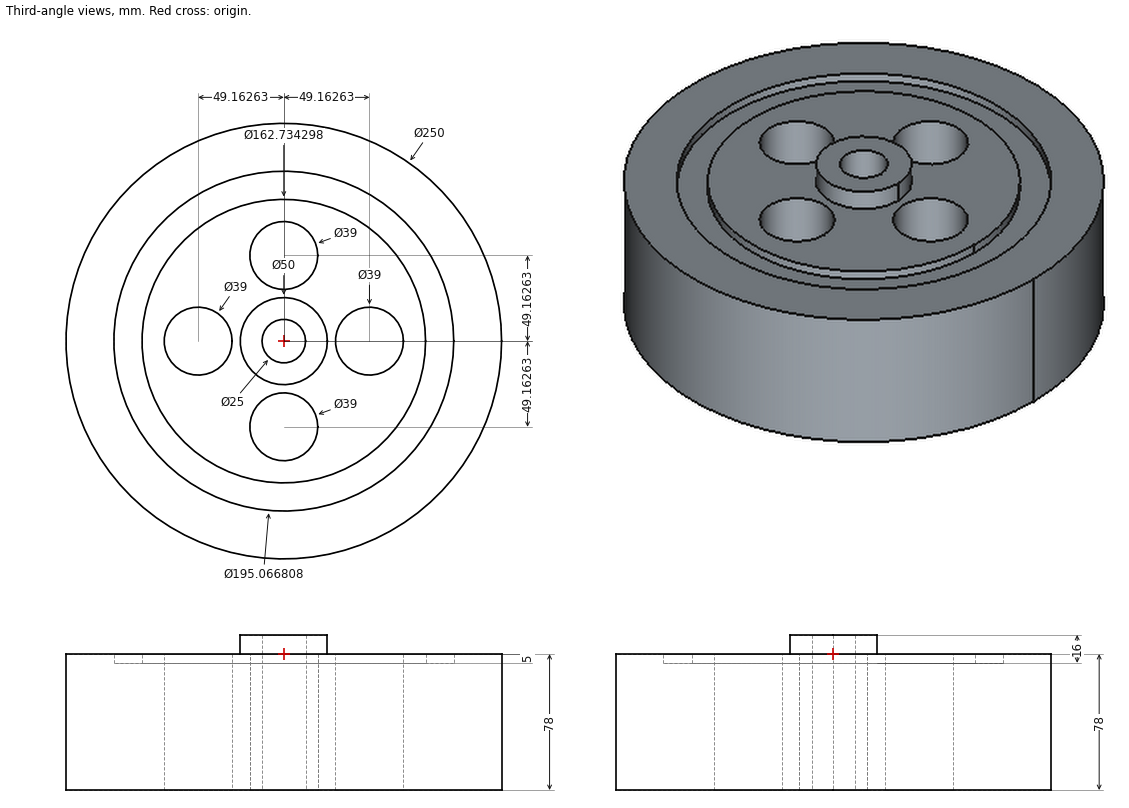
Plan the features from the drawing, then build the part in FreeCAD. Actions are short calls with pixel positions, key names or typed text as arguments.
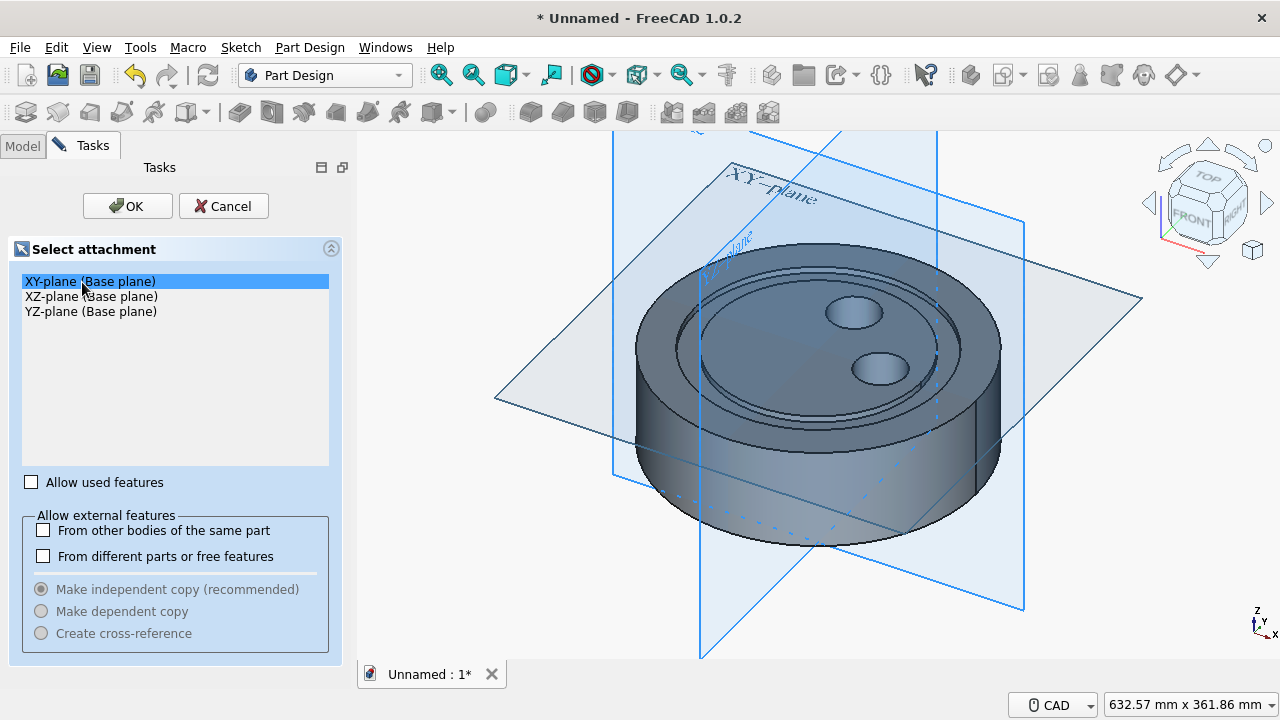
click(128, 206)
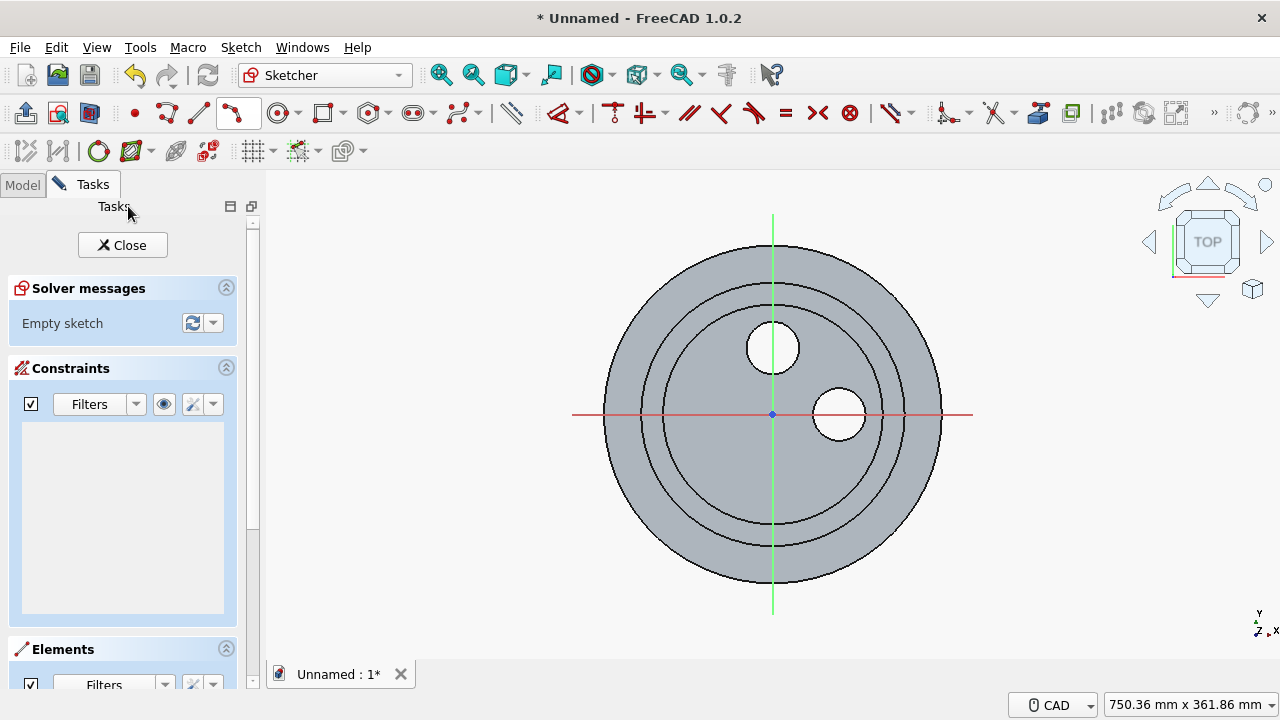
scroll(802, 481, up, 6)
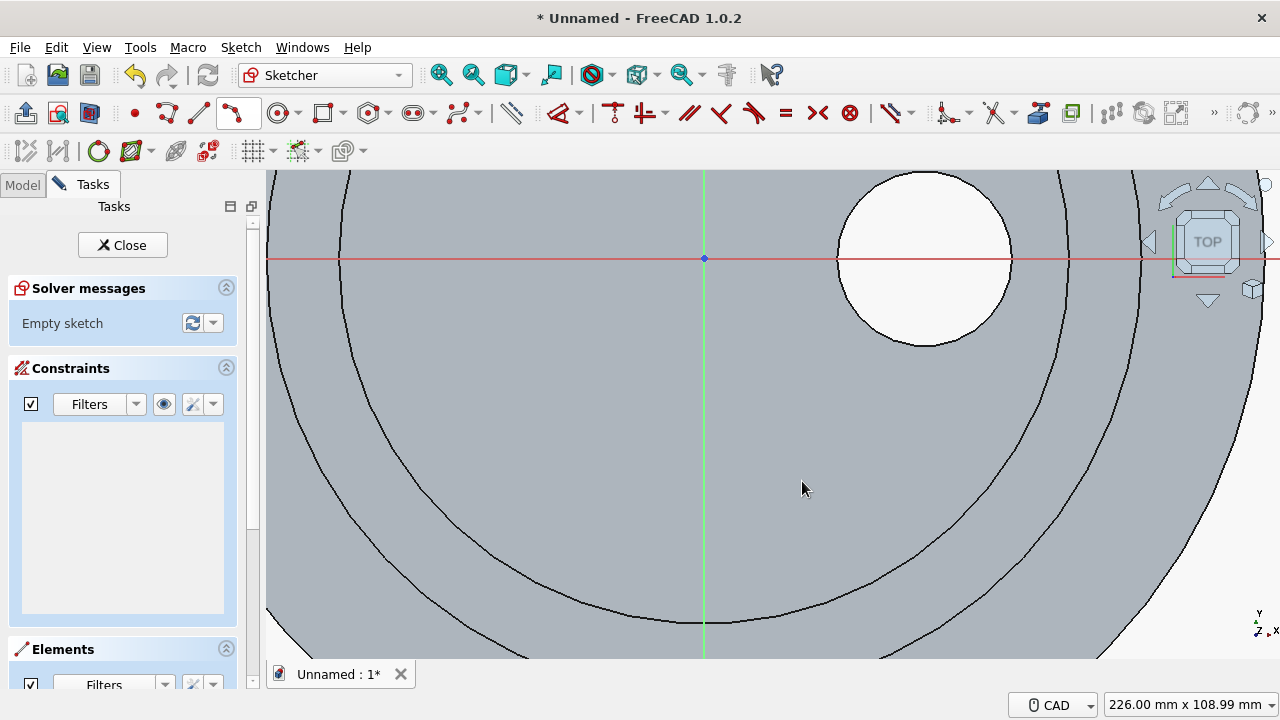
key(g)
key(c)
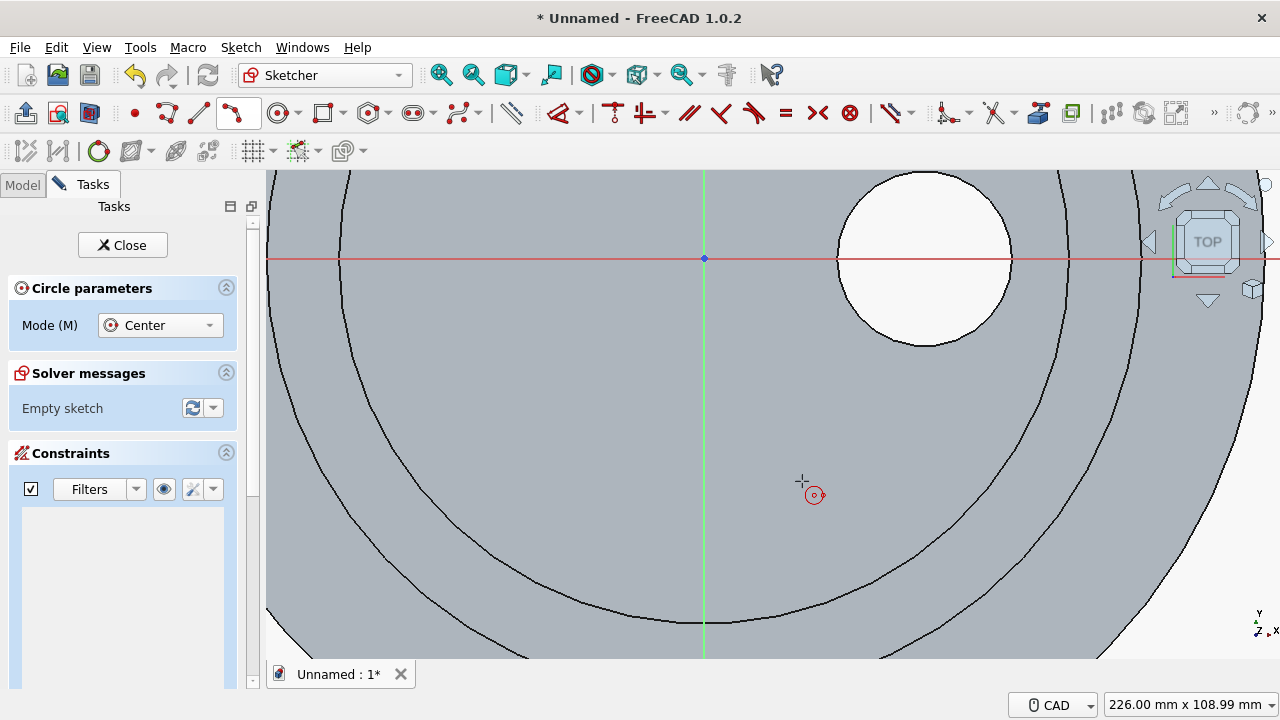
click(704, 479)
move(766, 417)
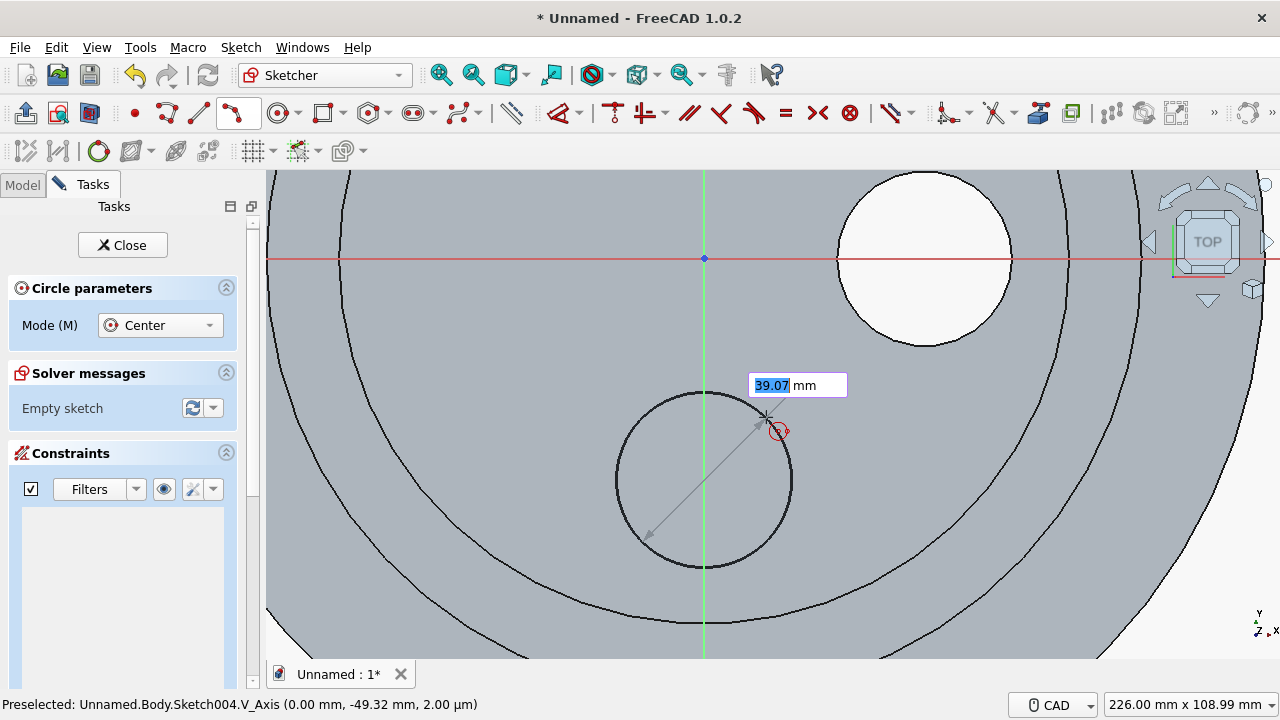
text(39)
key(Return)
key(Escape)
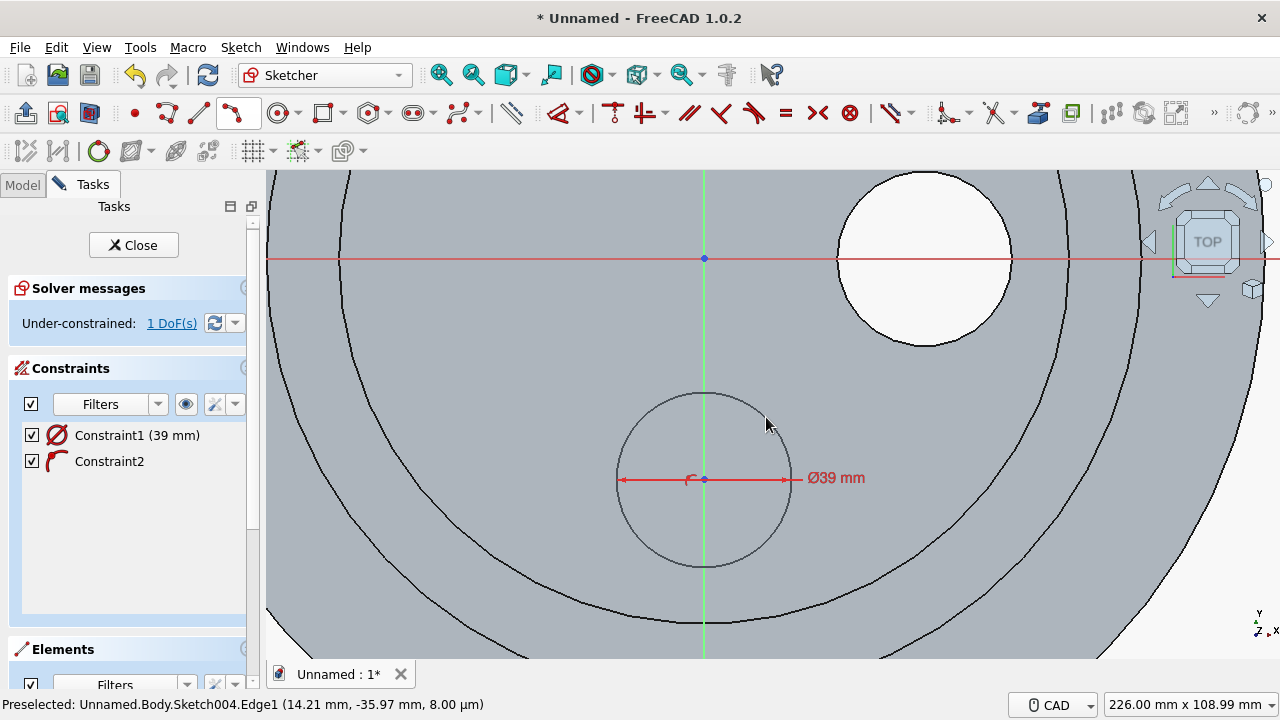
click(558, 114)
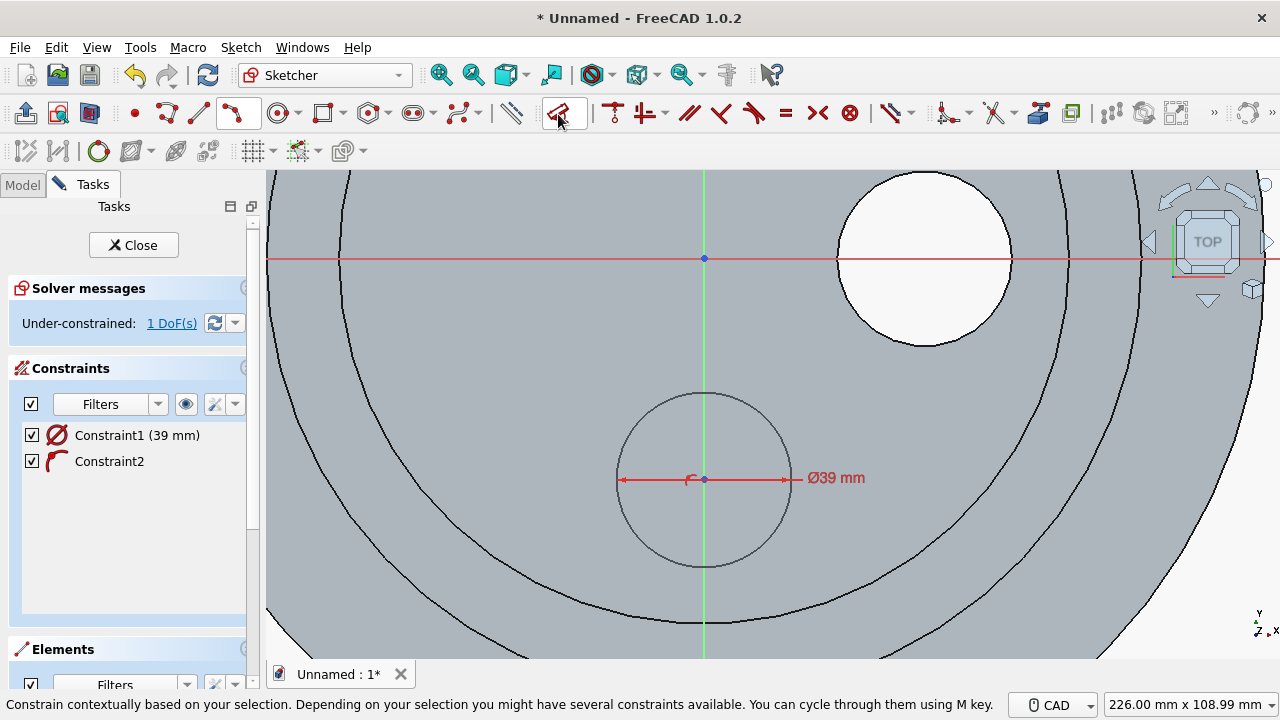
click(704, 480)
click(738, 369)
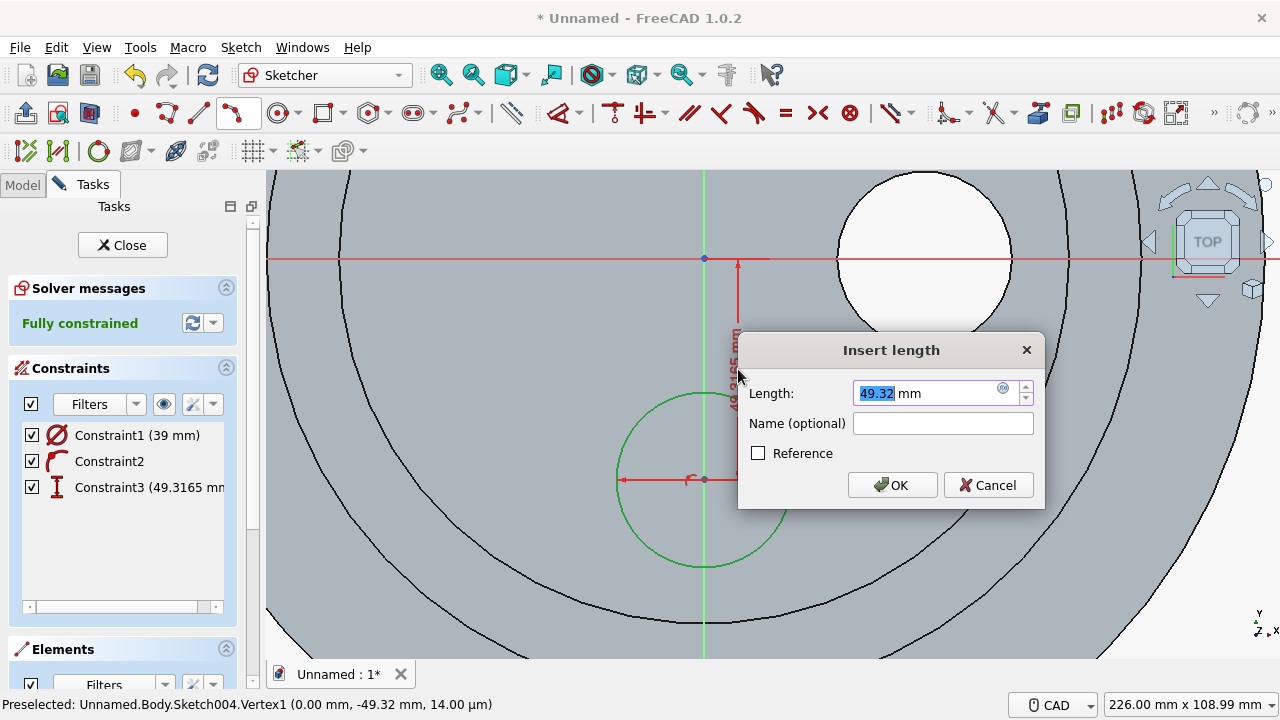
text(49.16263)
key(Return)
key(Escape)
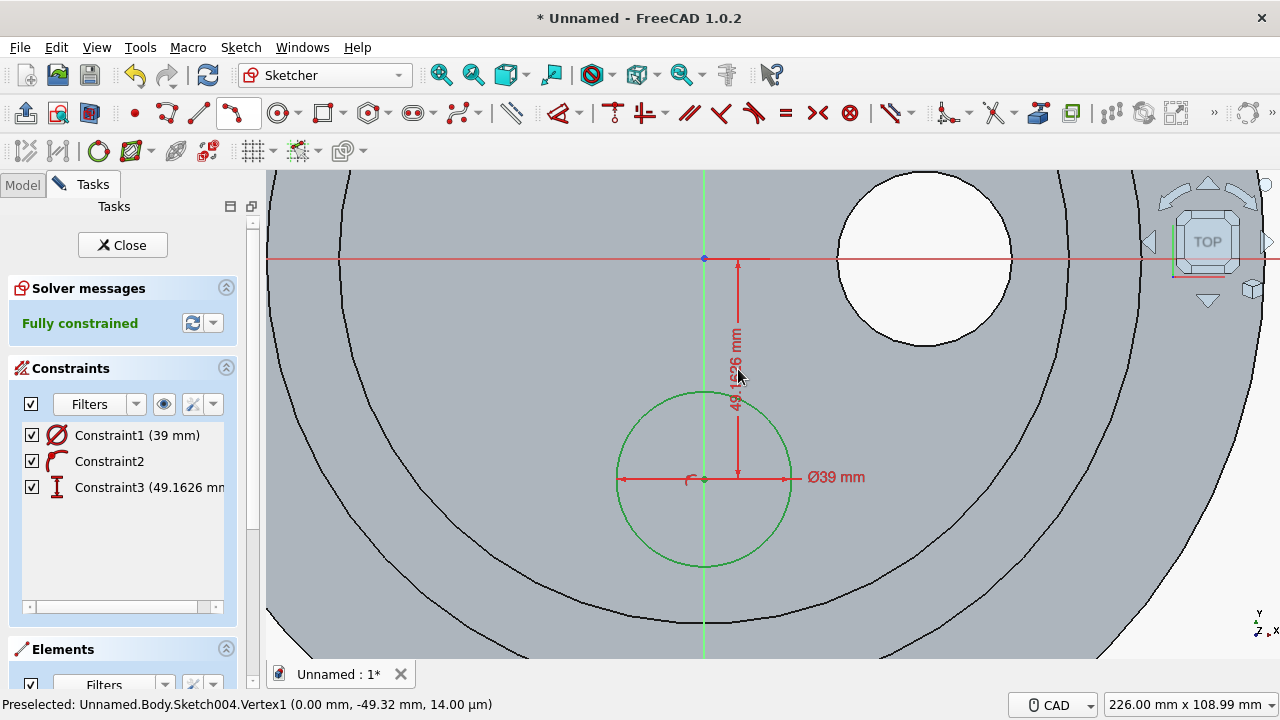
click(123, 245)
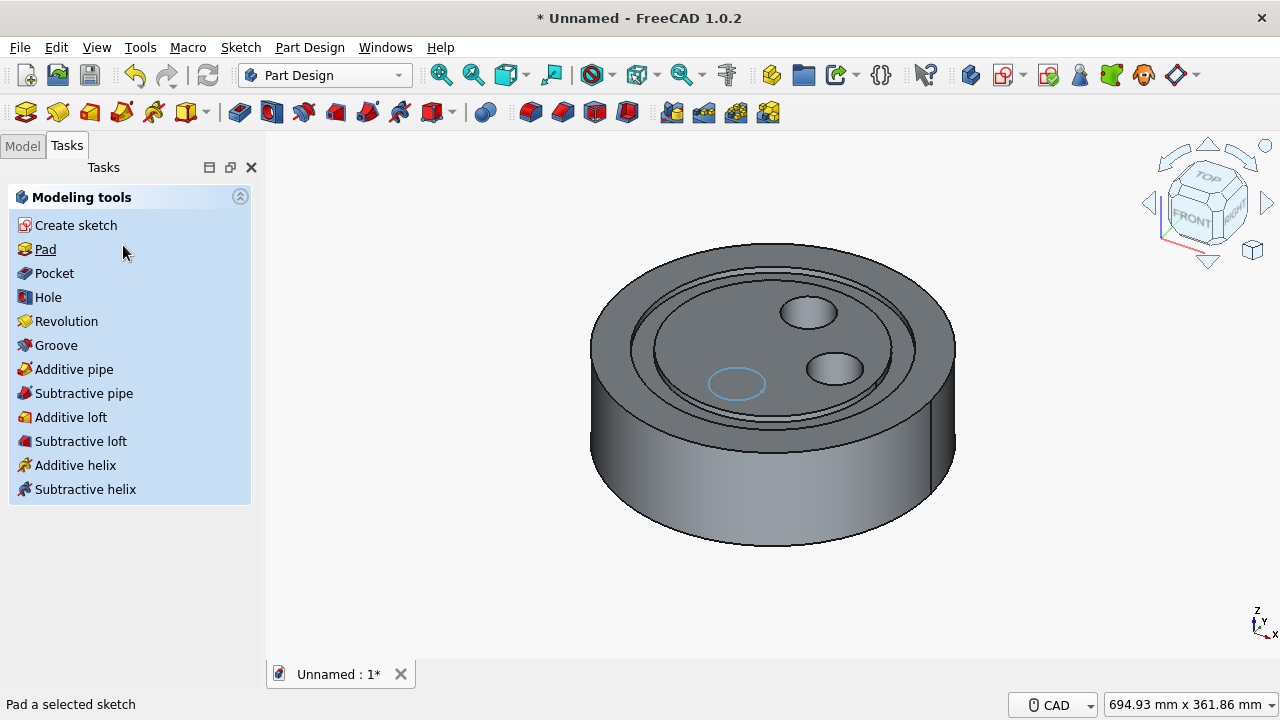
click(240, 112)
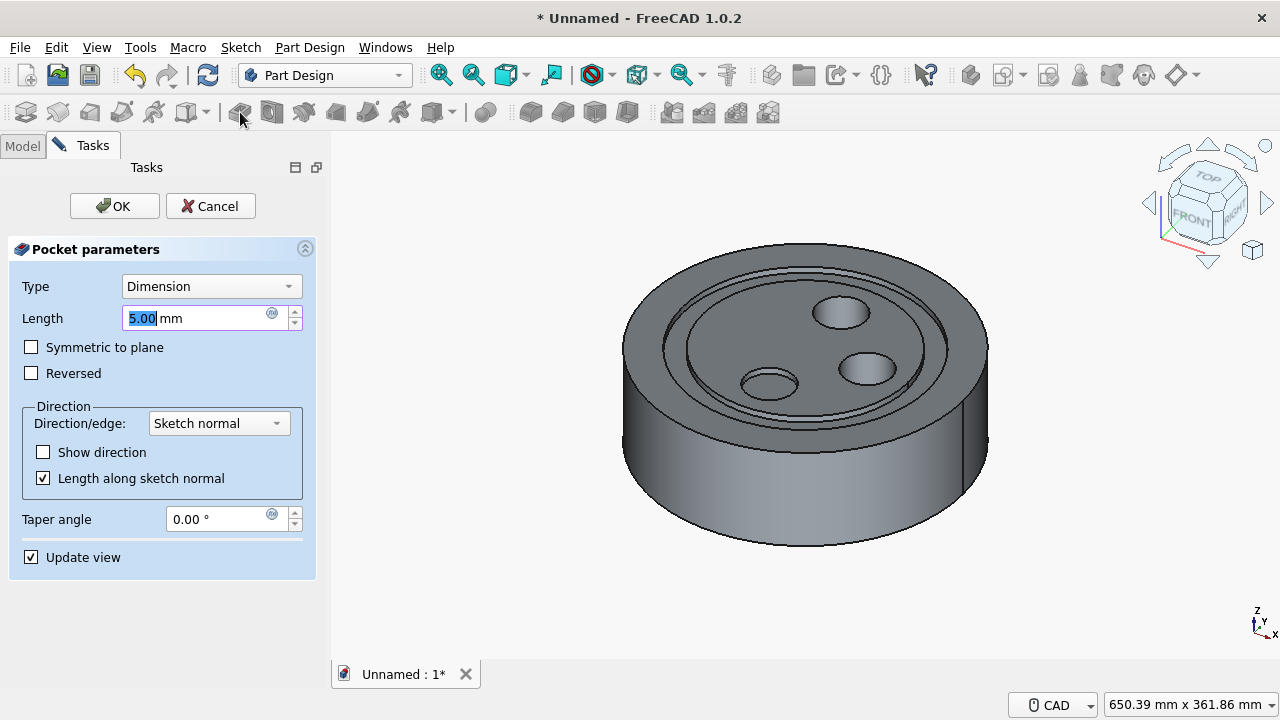
text(78)
key(Tab)